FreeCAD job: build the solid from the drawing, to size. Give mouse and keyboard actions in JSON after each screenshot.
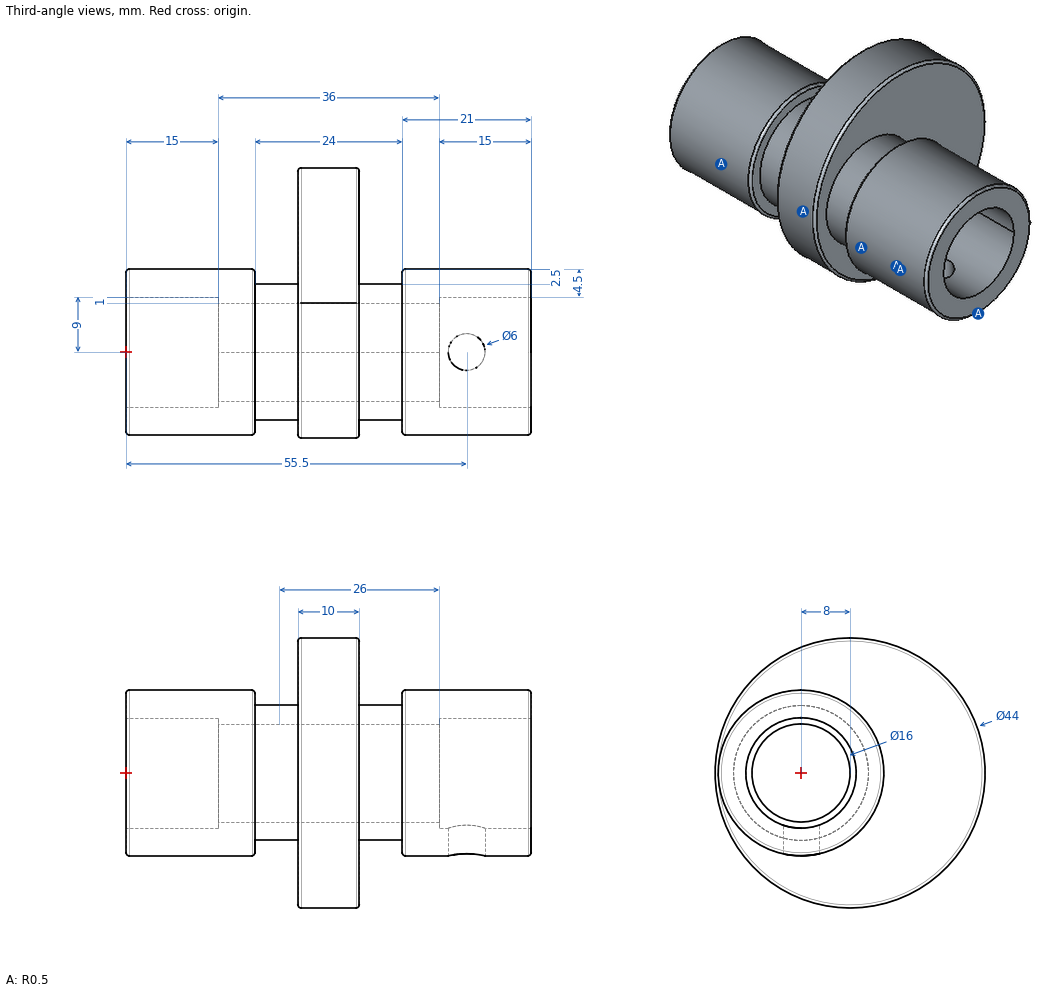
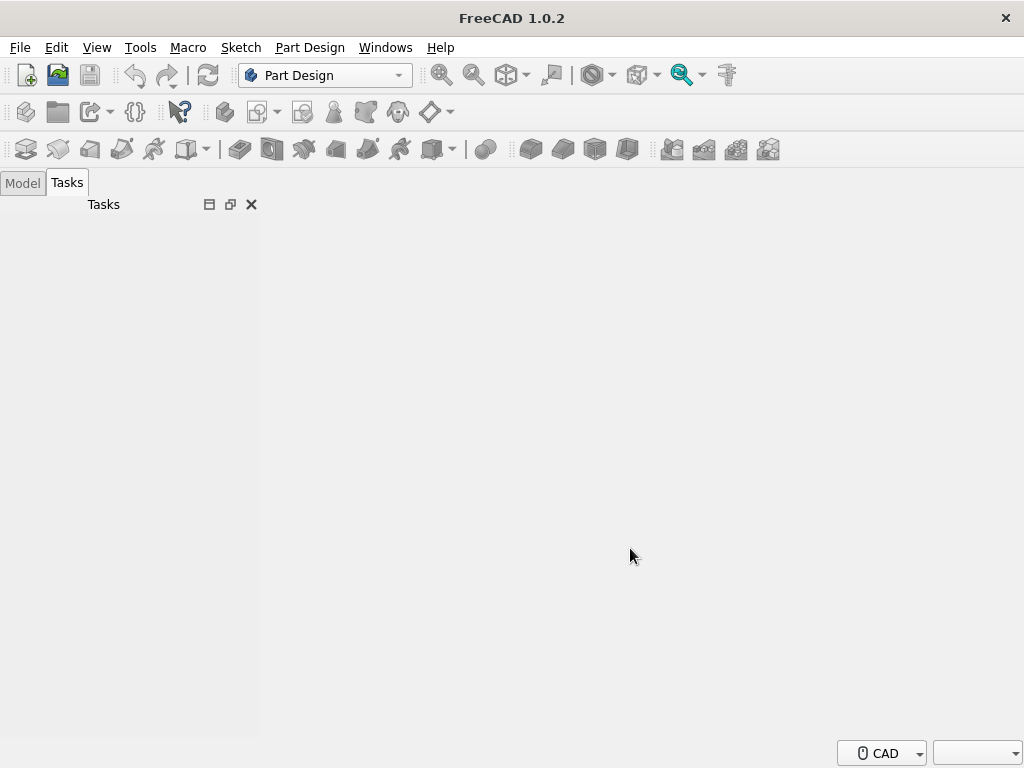
{"action": "left_click", "coordinate": [26, 76]}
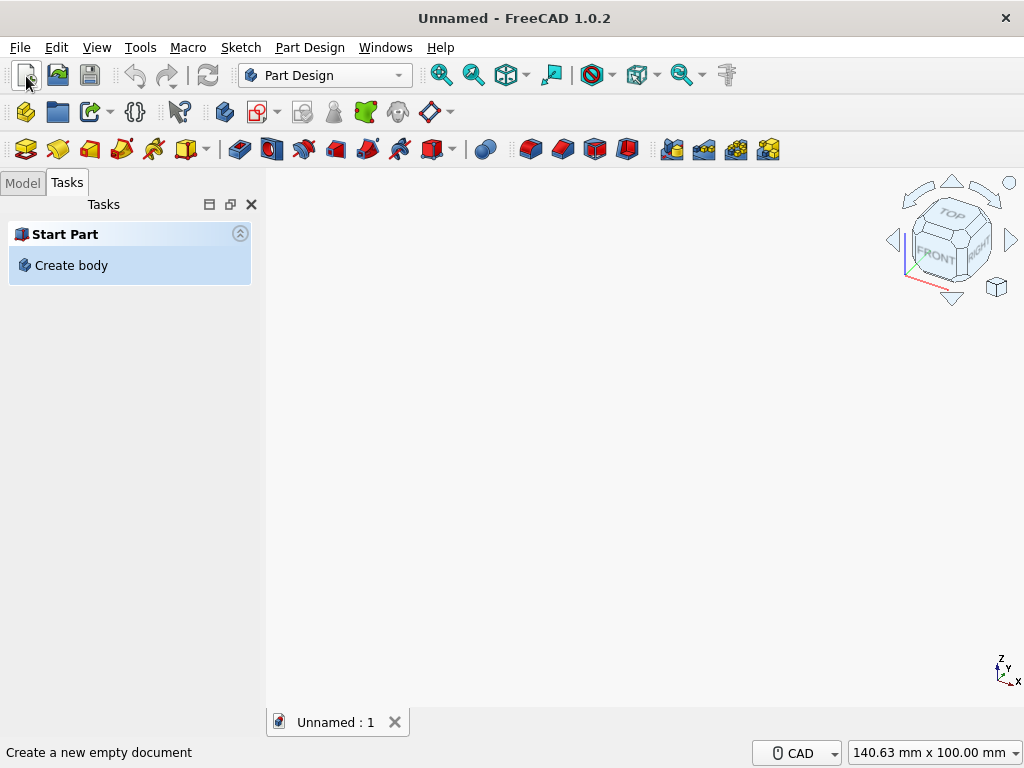
{"action": "left_click", "coordinate": [258, 112]}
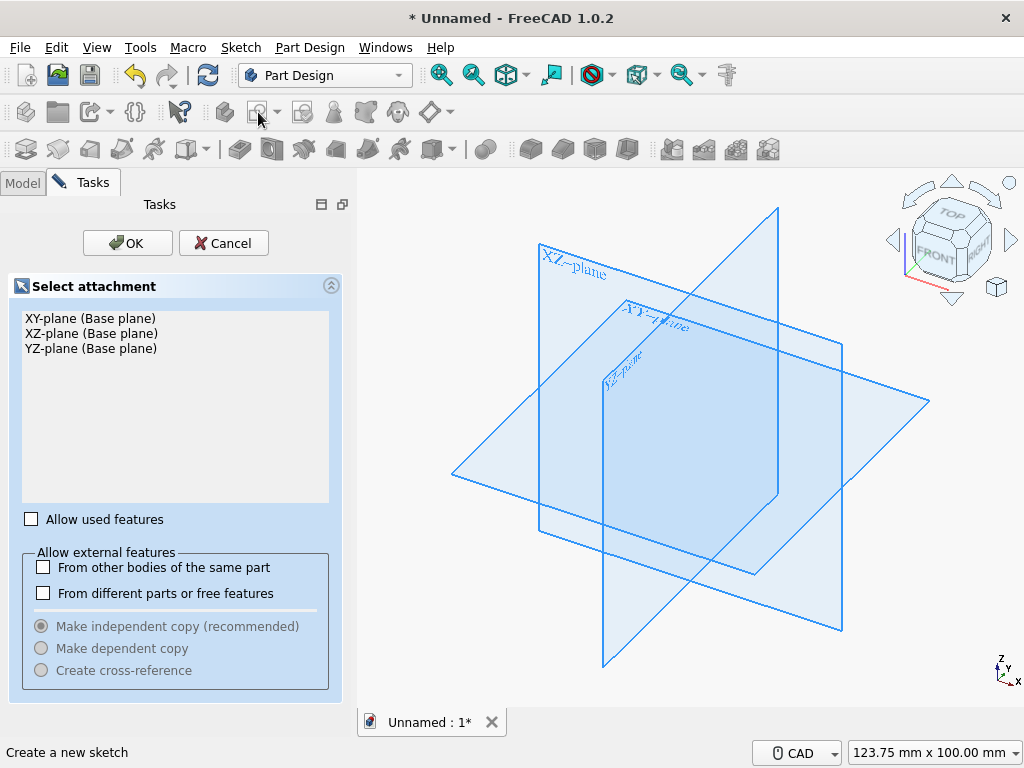
{"action": "left_click", "coordinate": [82, 318]}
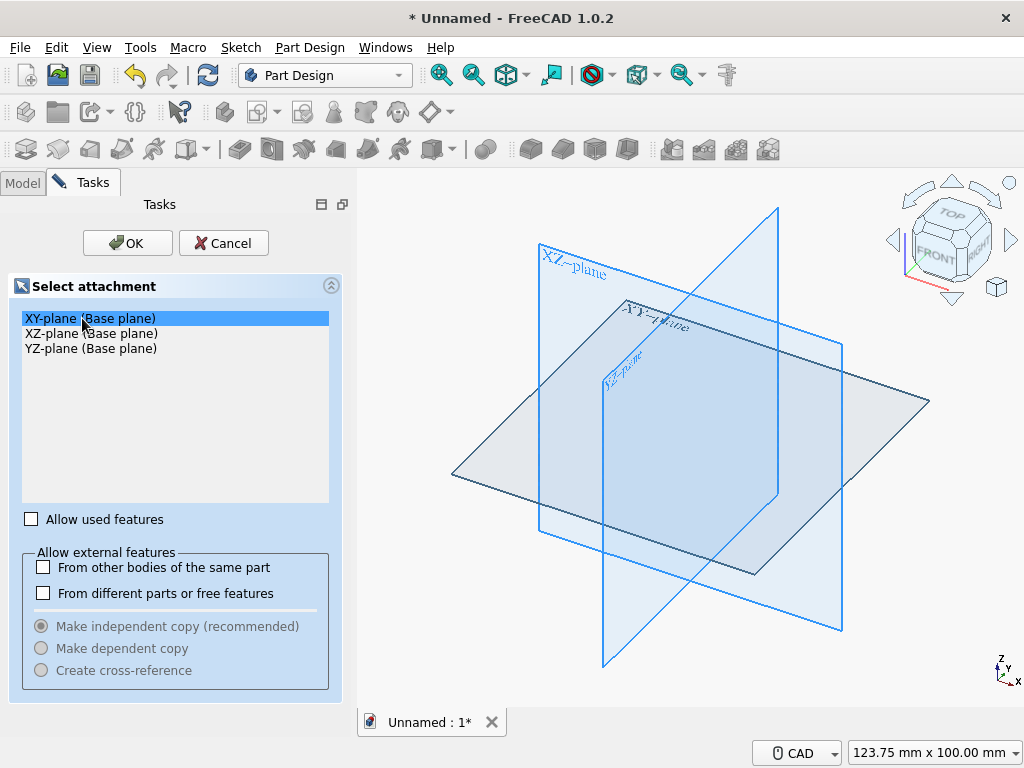
{"action": "left_click", "coordinate": [128, 243]}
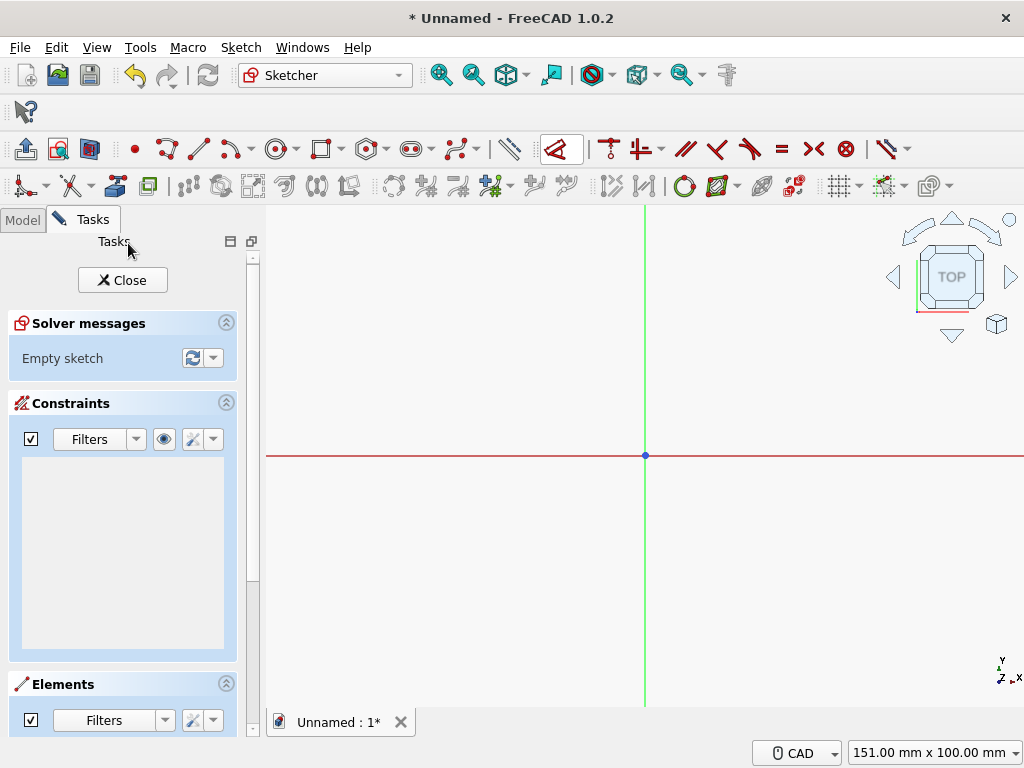
{"action": "scroll", "coordinate": [294, 525], "scroll_direction": "down", "scroll_amount": 2}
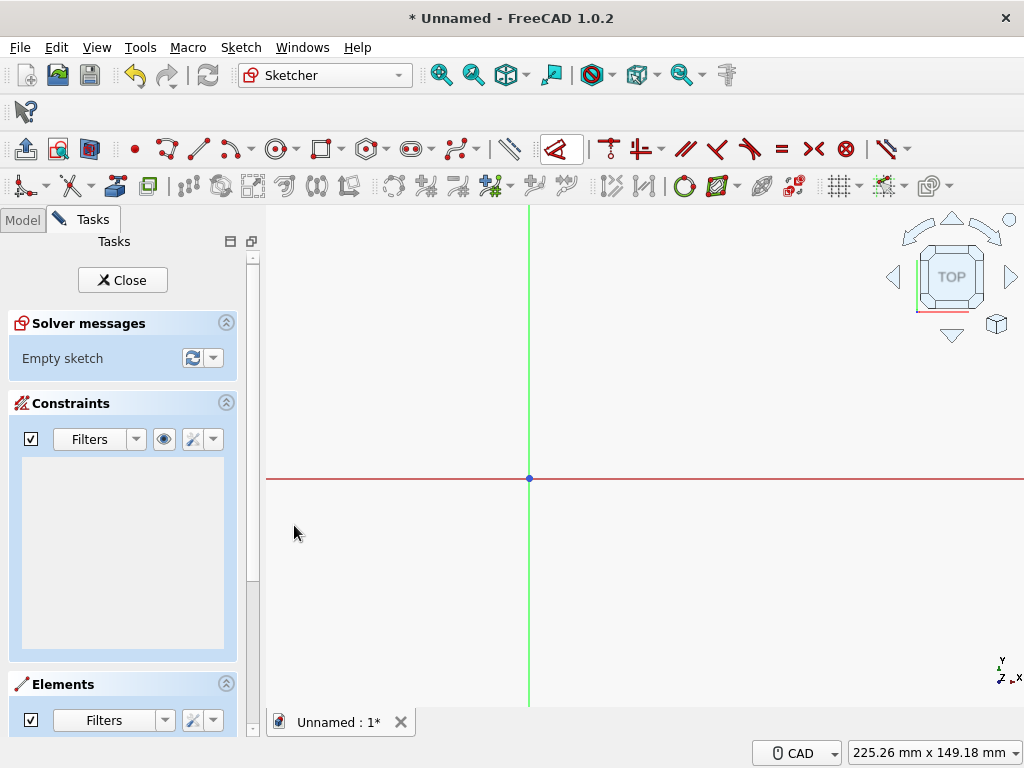
{"action": "scroll", "coordinate": [718, 457], "scroll_direction": "up", "scroll_amount": 3}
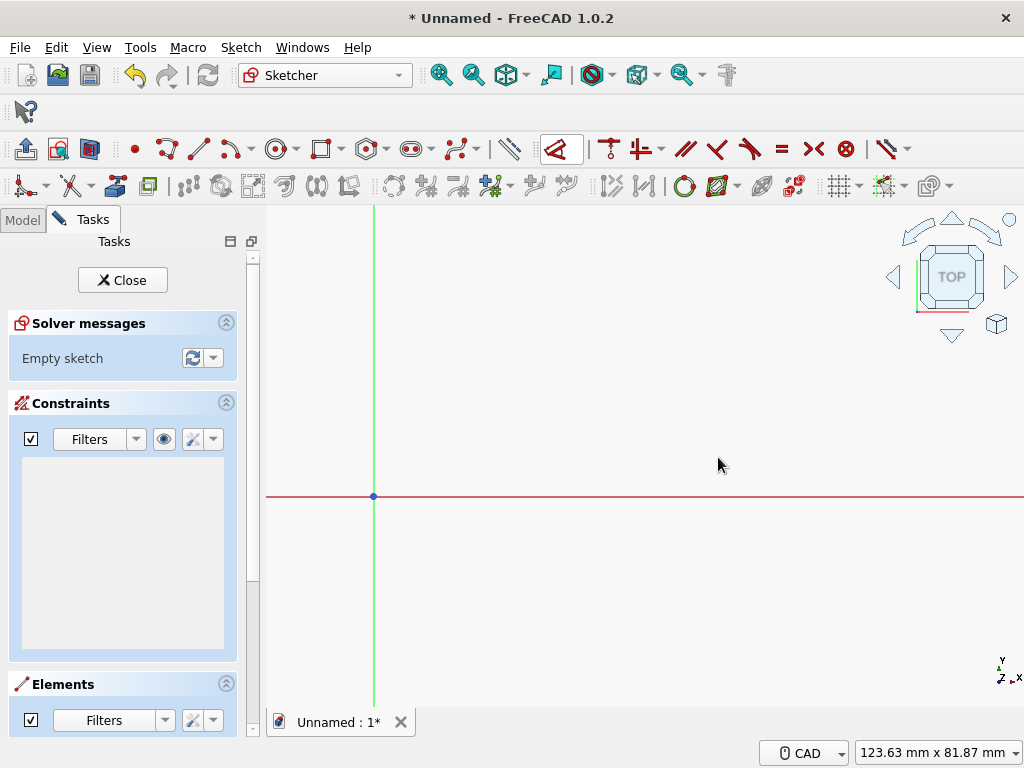
{"action": "left_click", "coordinate": [168, 150]}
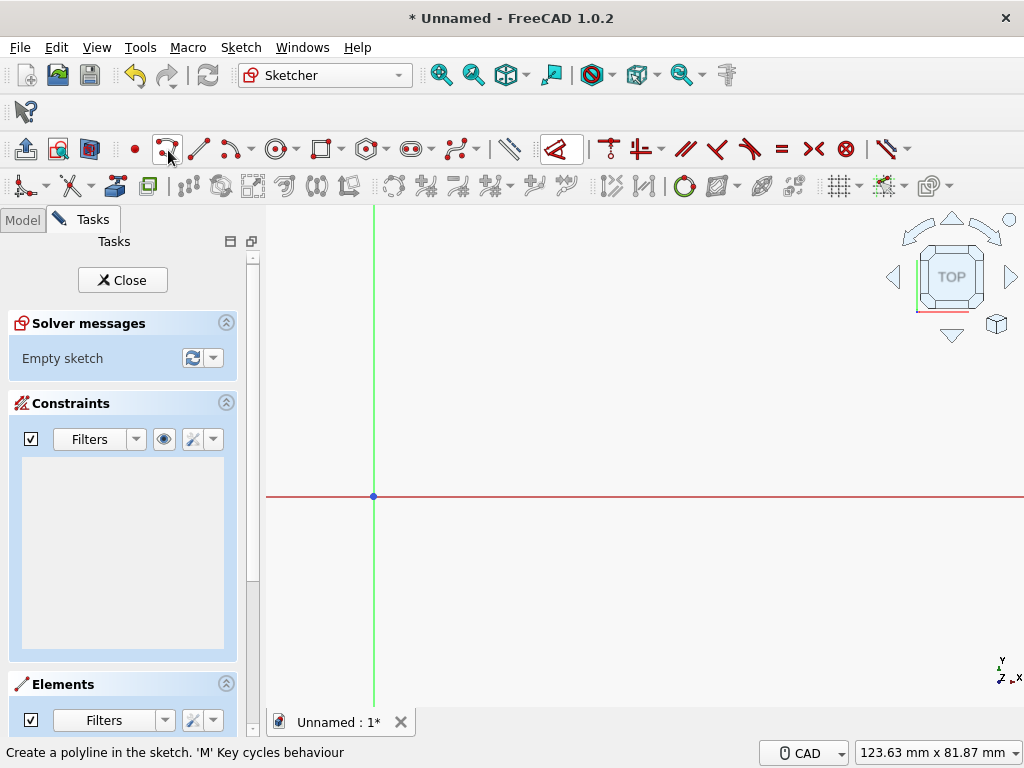
{"action": "left_click", "coordinate": [374, 441]}
{"action": "left_click", "coordinate": [466, 441]}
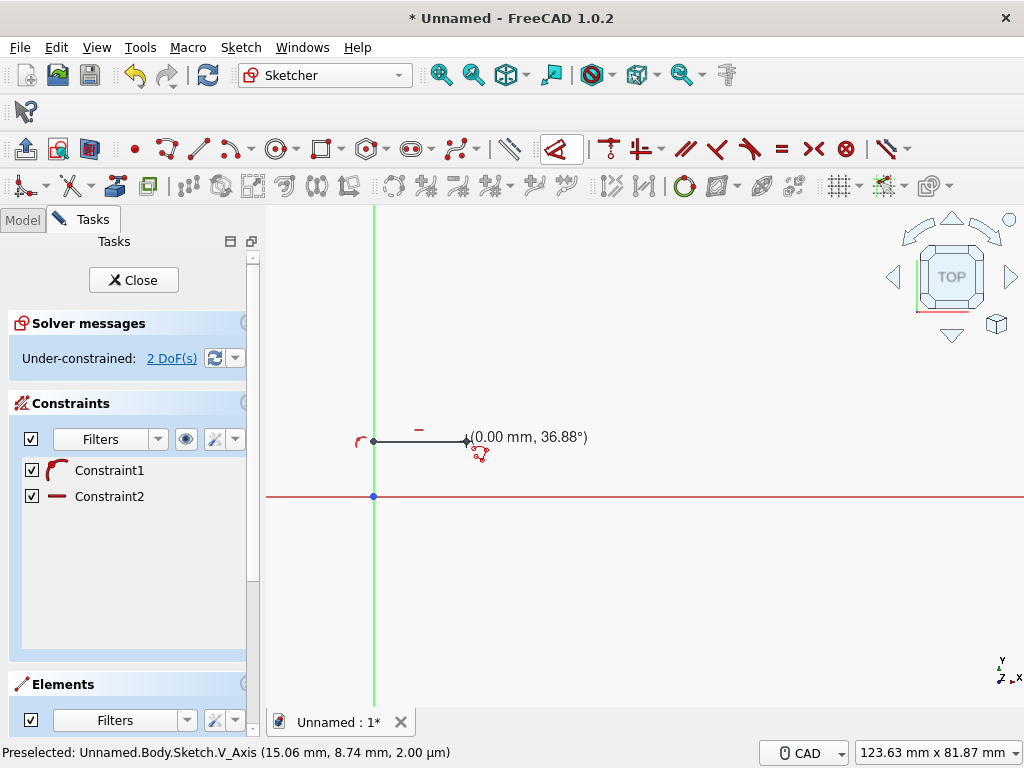
{"action": "scroll", "coordinate": [466, 448], "scroll_direction": "up", "scroll_amount": 5}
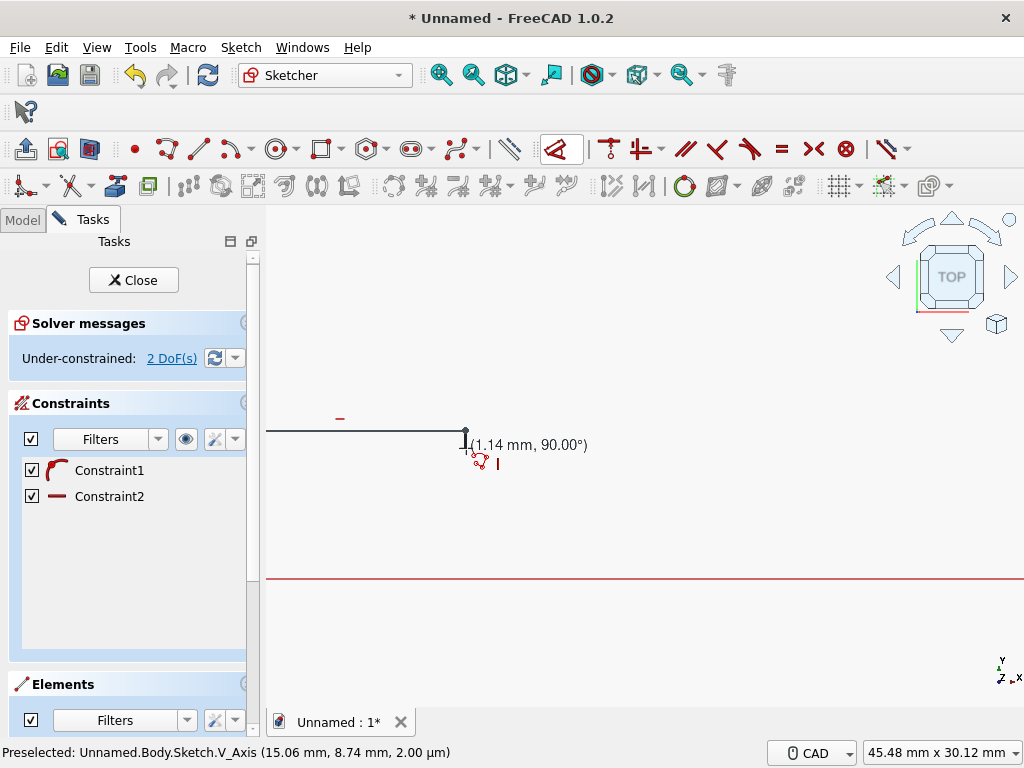
{"action": "left_click", "coordinate": [466, 446]}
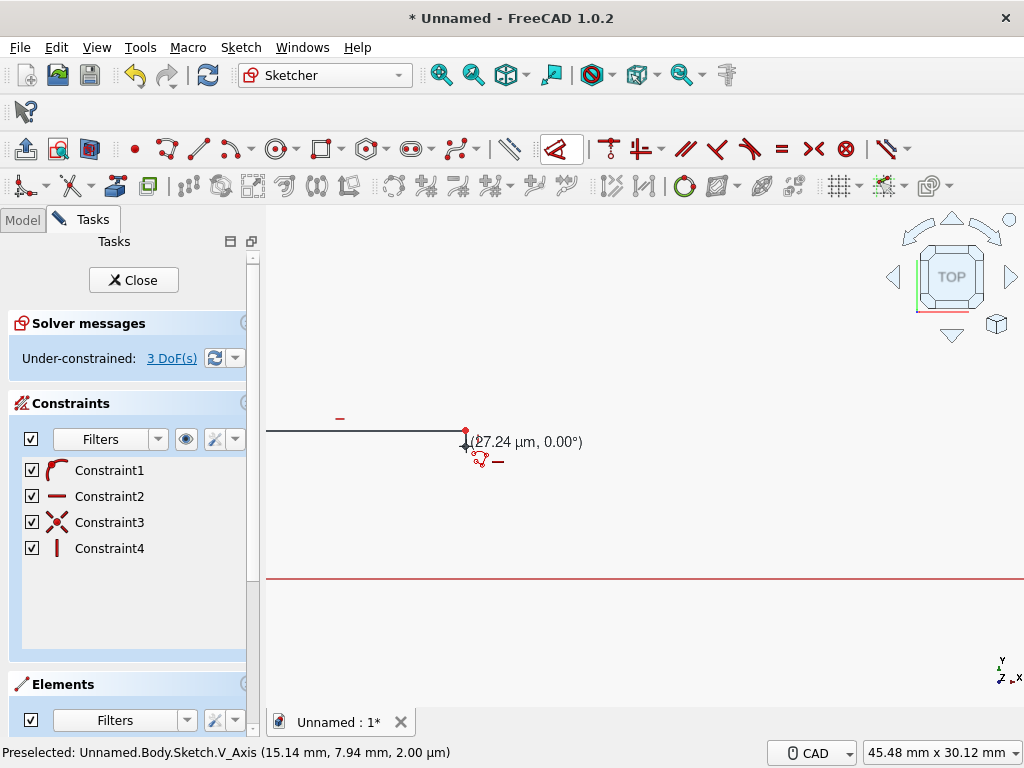
{"action": "scroll", "coordinate": [467, 450], "scroll_direction": "down", "scroll_amount": 5}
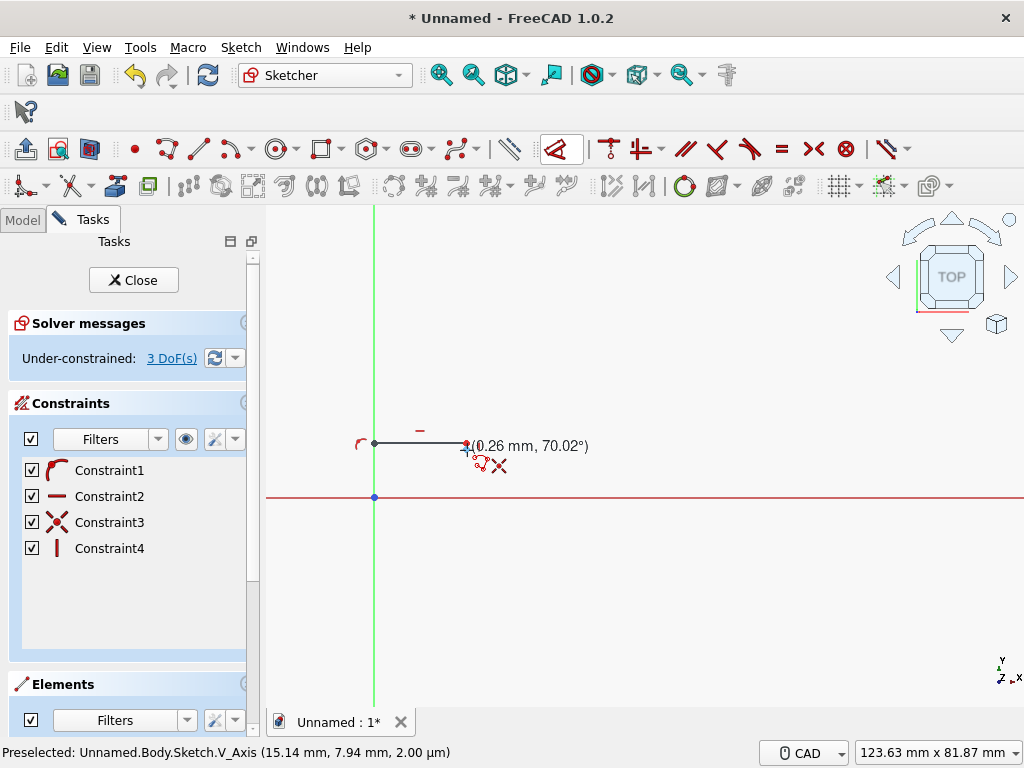
{"action": "left_click", "coordinate": [687, 449]}